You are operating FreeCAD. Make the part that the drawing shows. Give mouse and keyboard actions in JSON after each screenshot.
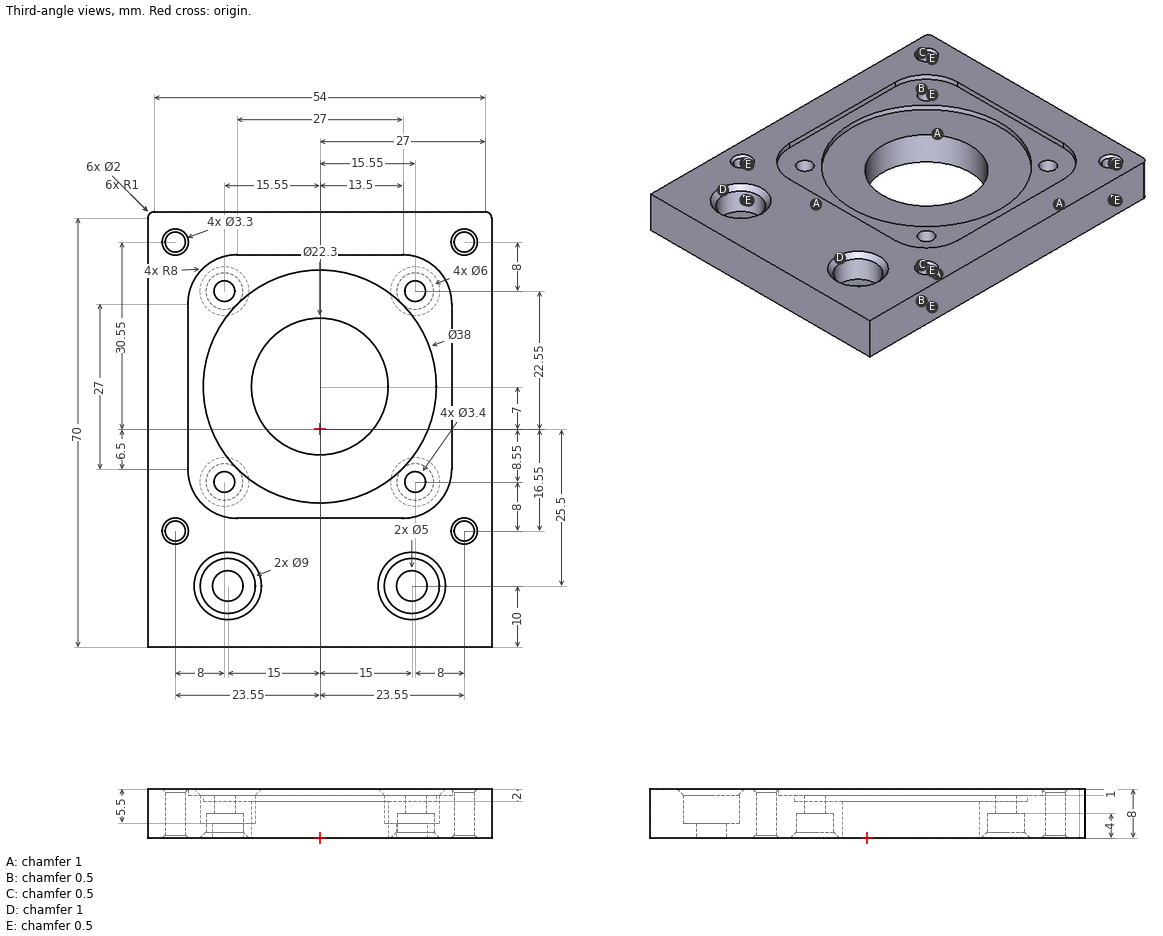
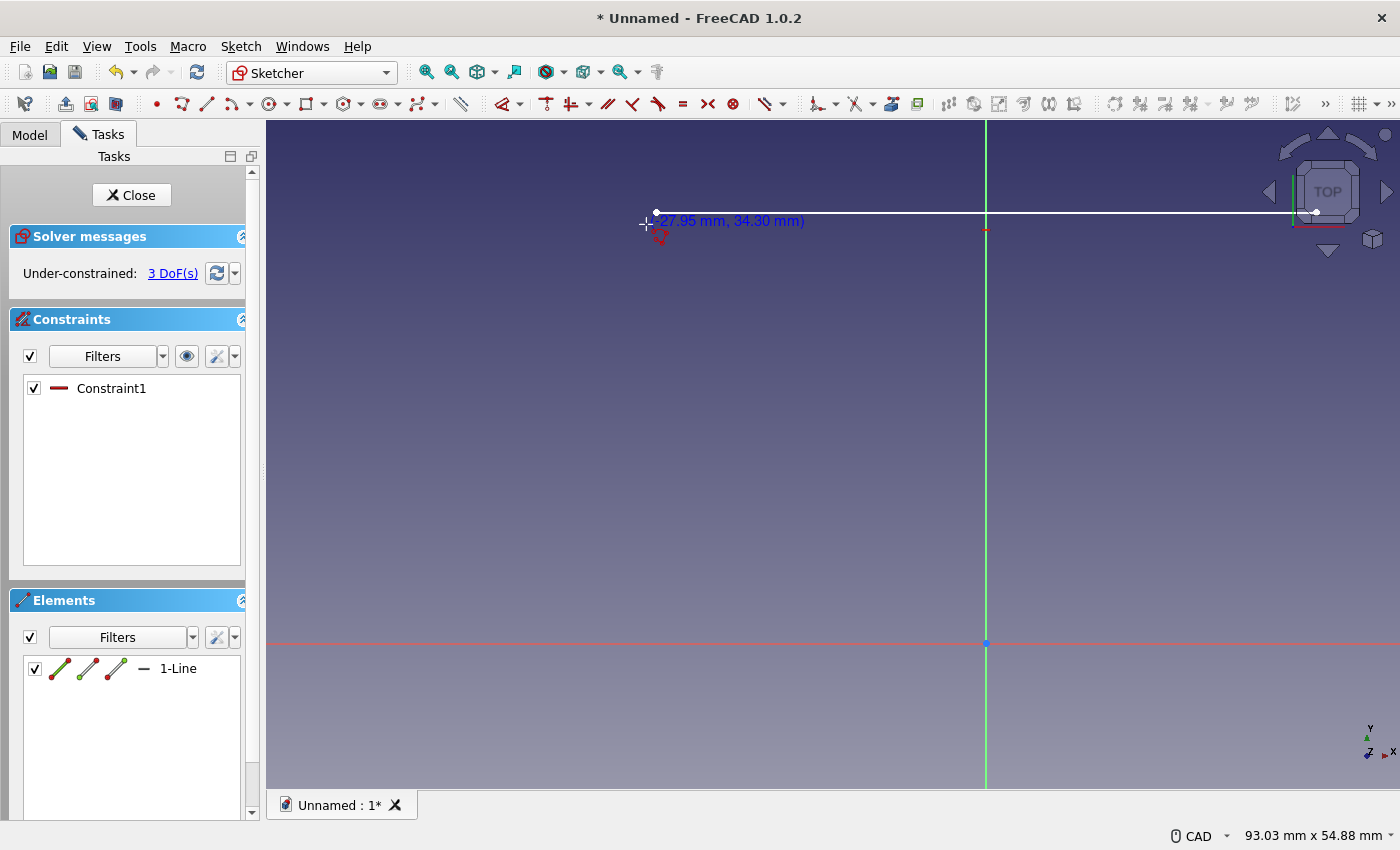
{"action": "left_click", "coordinate": [645, 223]}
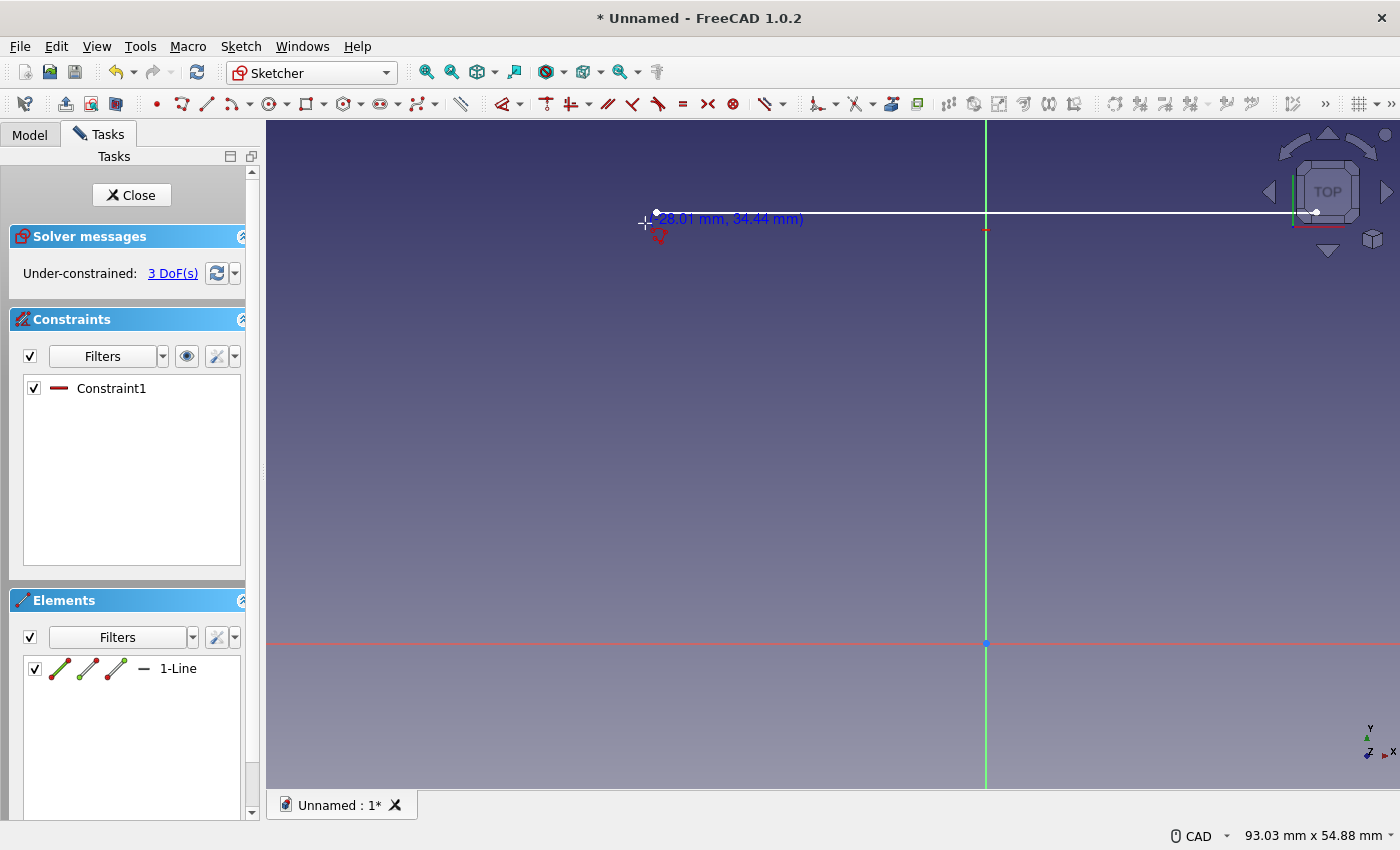
{"action": "scroll", "coordinate": [495, 224], "scroll_direction": "down", "scroll_amount": 3}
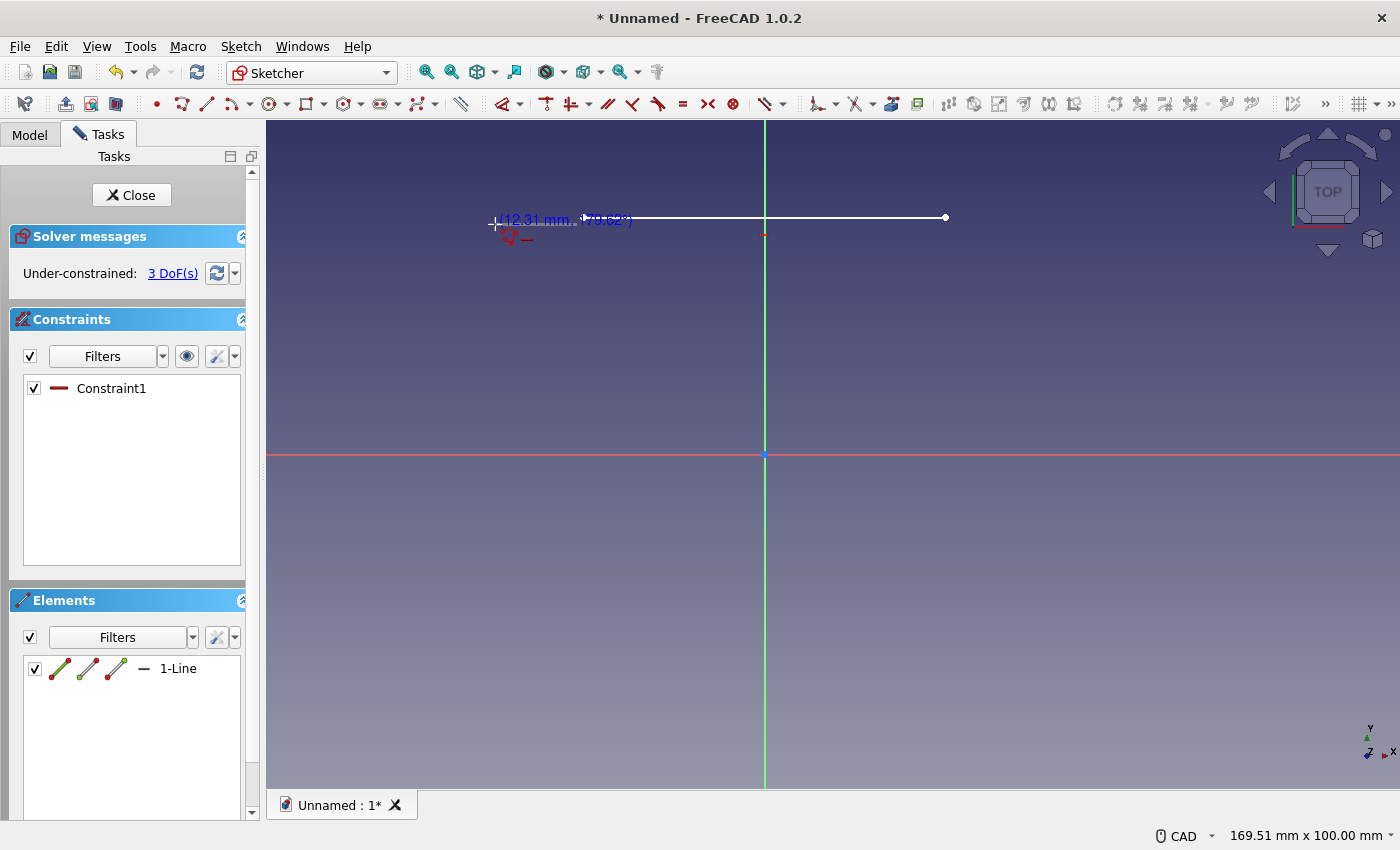
{"action": "left_click", "coordinate": [577, 692]}
{"action": "left_click", "coordinate": [952, 692]}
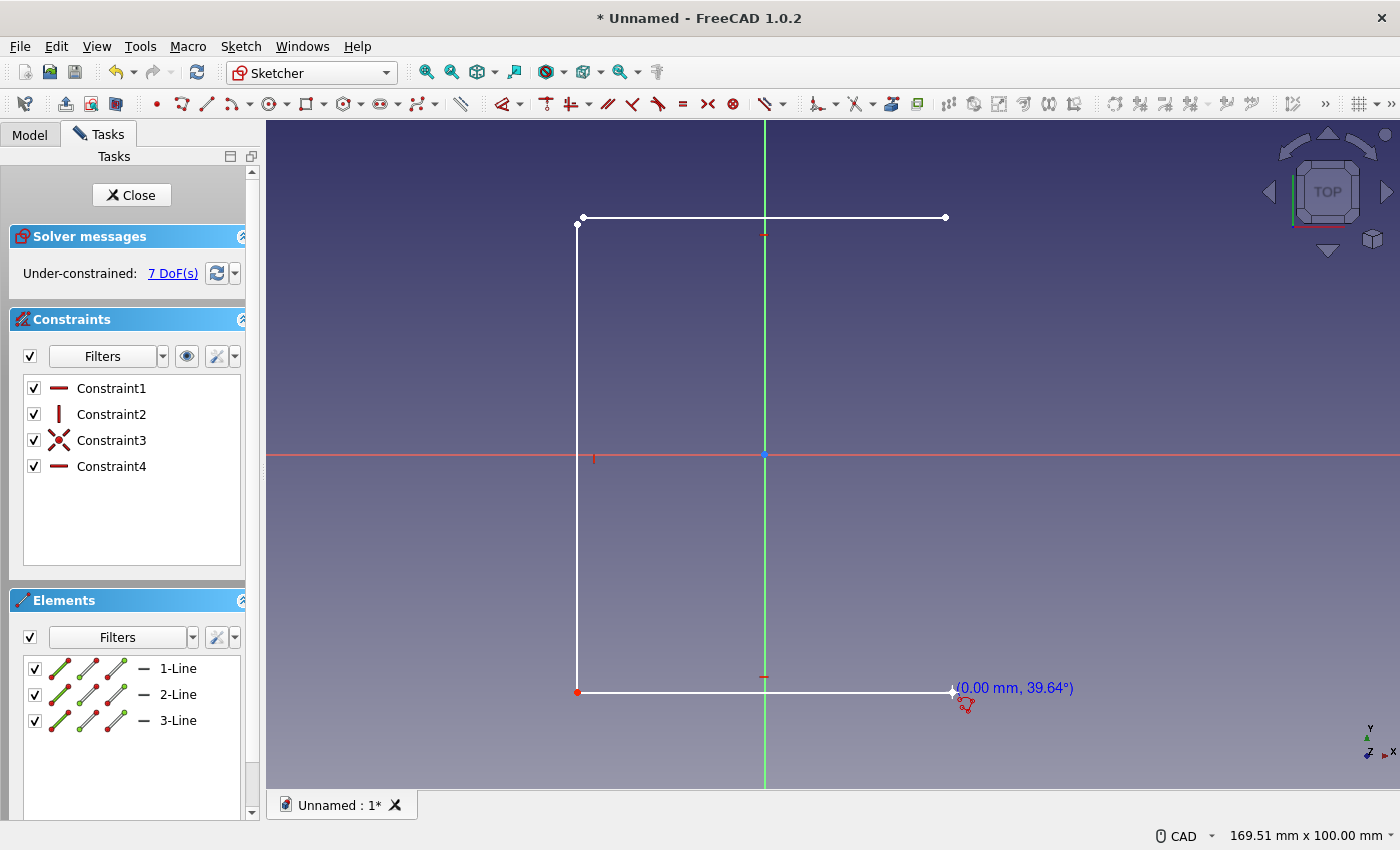
{"action": "scroll", "coordinate": [952, 224], "scroll_direction": "up", "scroll_amount": 3}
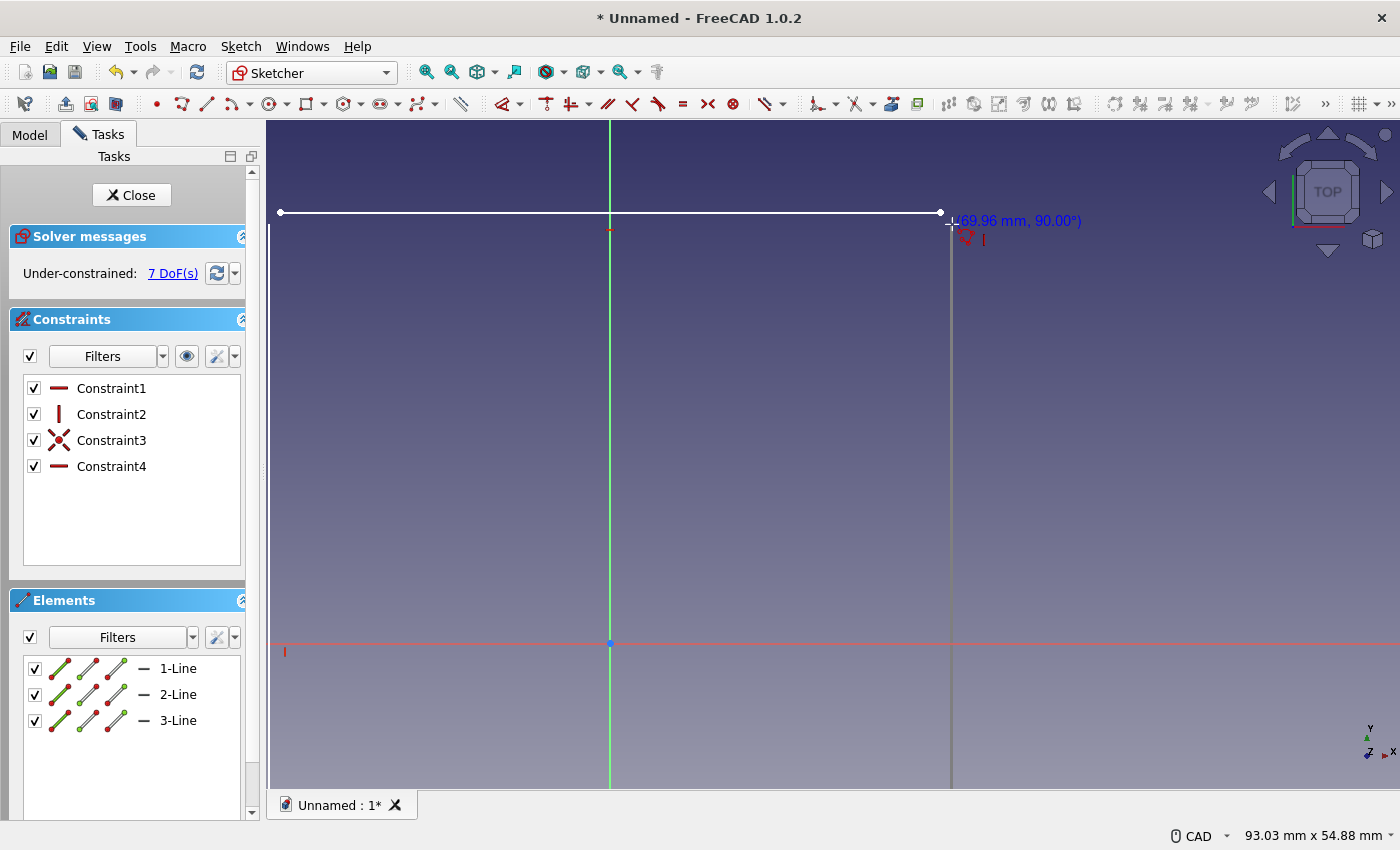
{"action": "left_click", "coordinate": [952, 223]}
{"action": "right_click", "coordinate": [952, 223]}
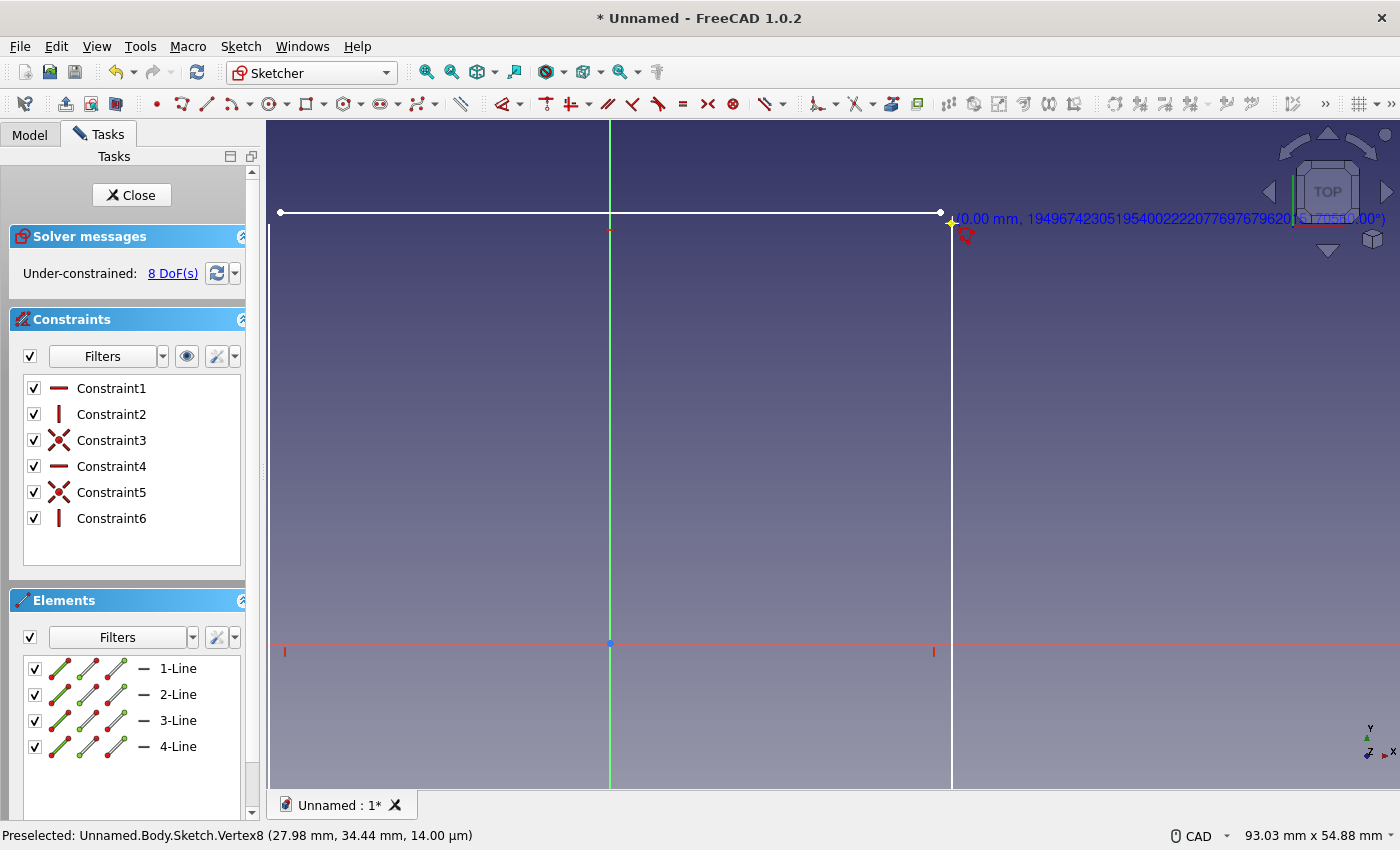
{"action": "left_click", "coordinate": [250, 104]}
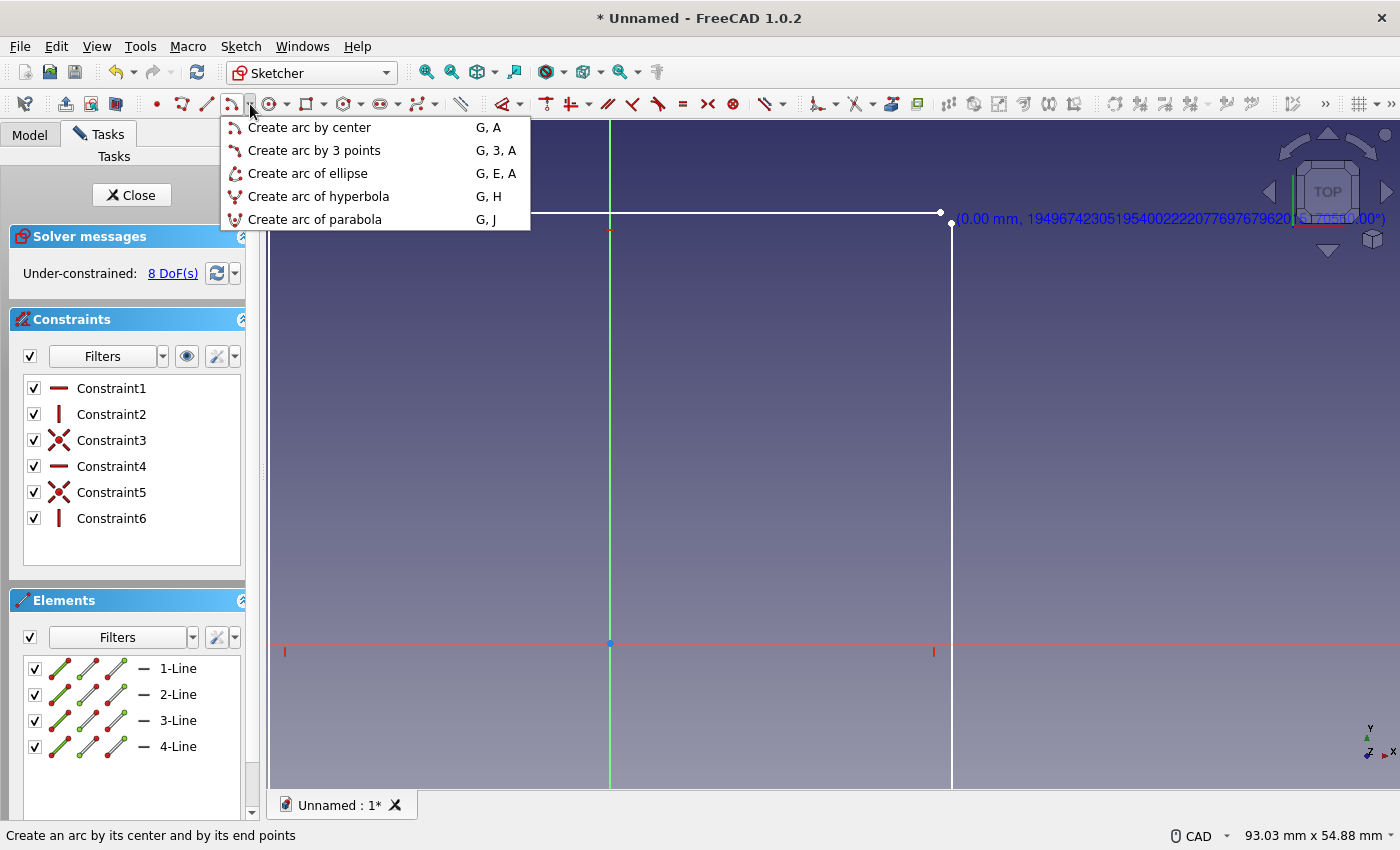
{"action": "left_click", "coordinate": [376, 150]}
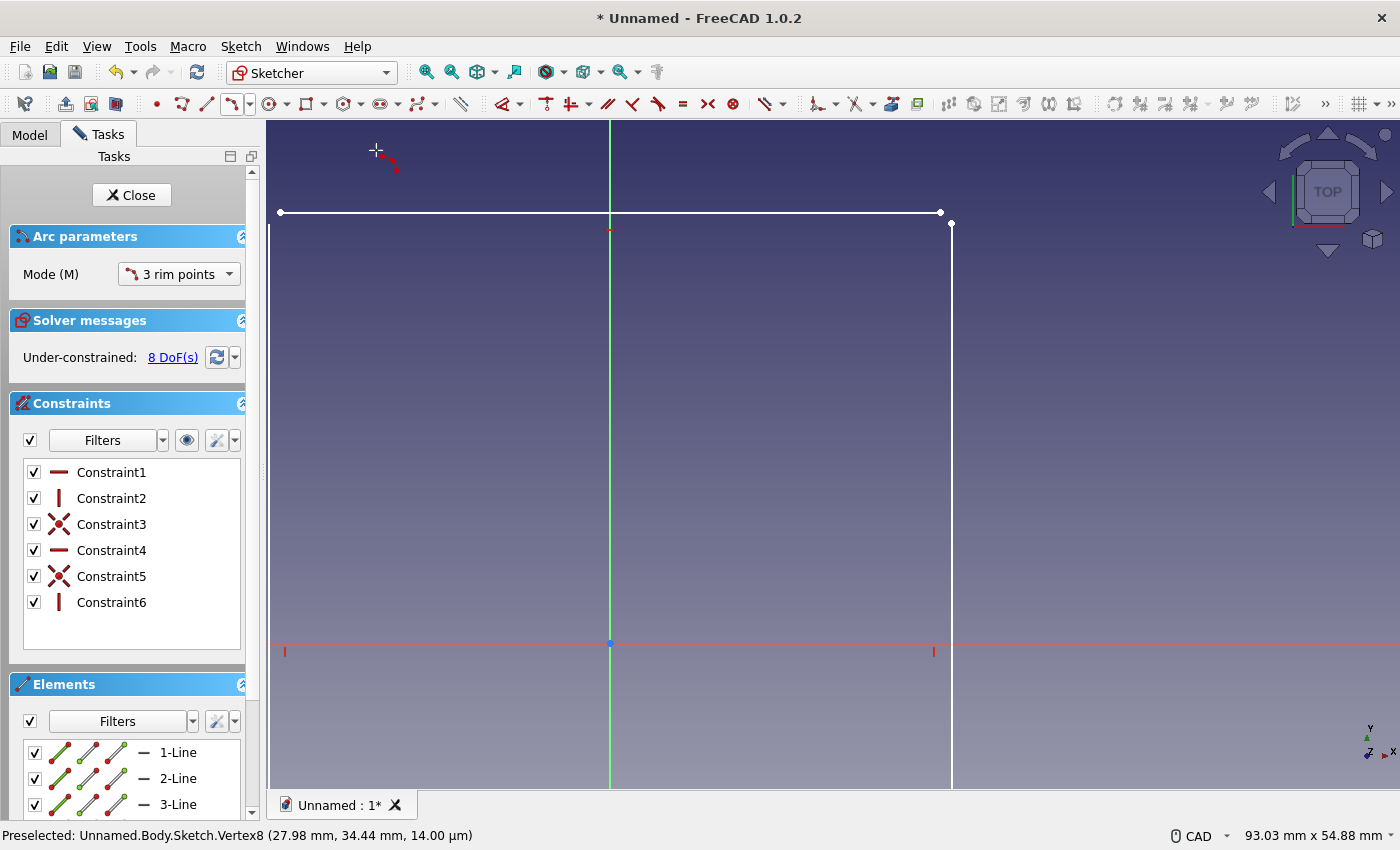
{"action": "scroll", "coordinate": [952, 224], "scroll_direction": "down", "scroll_amount": 3}